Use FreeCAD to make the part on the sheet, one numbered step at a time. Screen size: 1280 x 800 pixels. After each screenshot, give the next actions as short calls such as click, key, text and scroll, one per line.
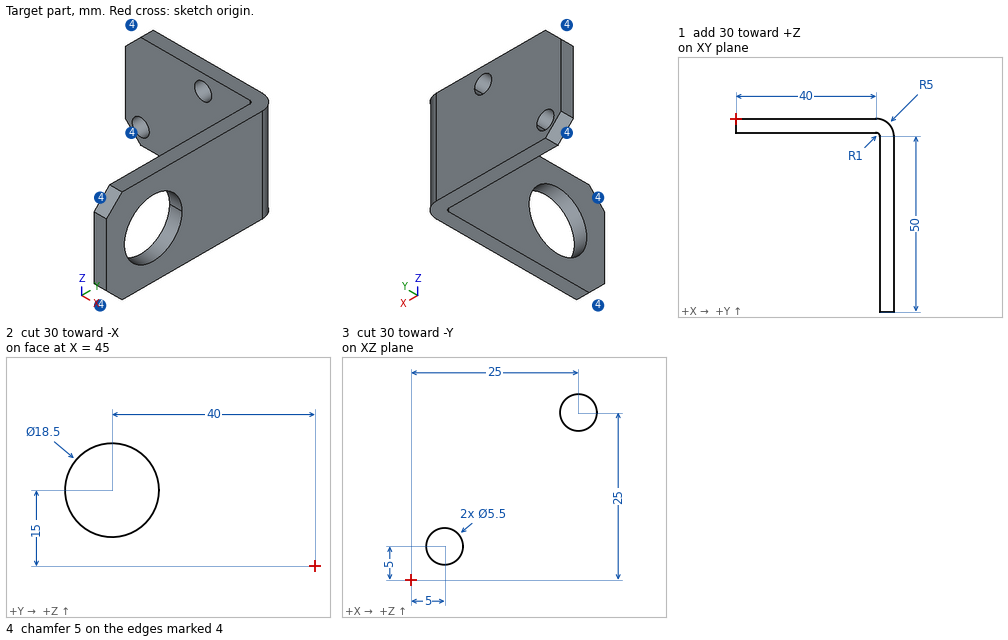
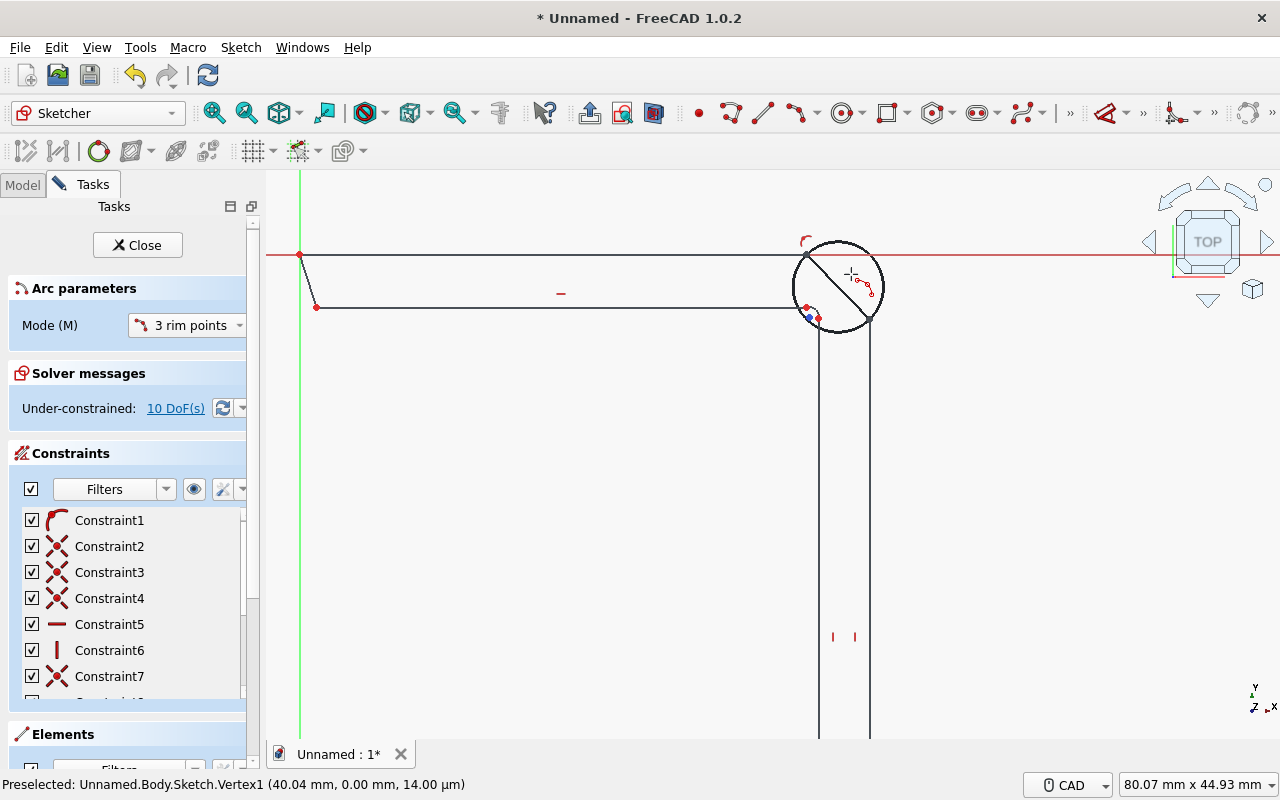
click(851, 273)
key(Escape)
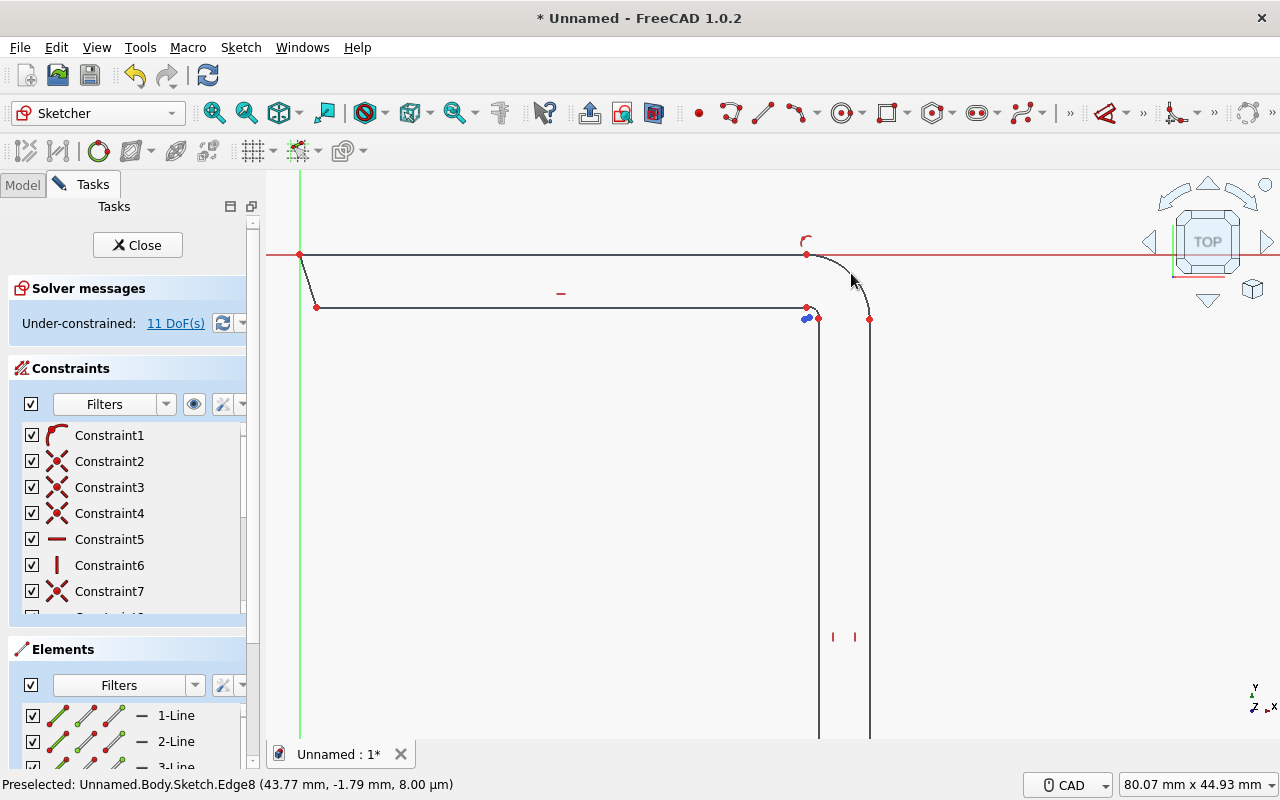
click(655, 255)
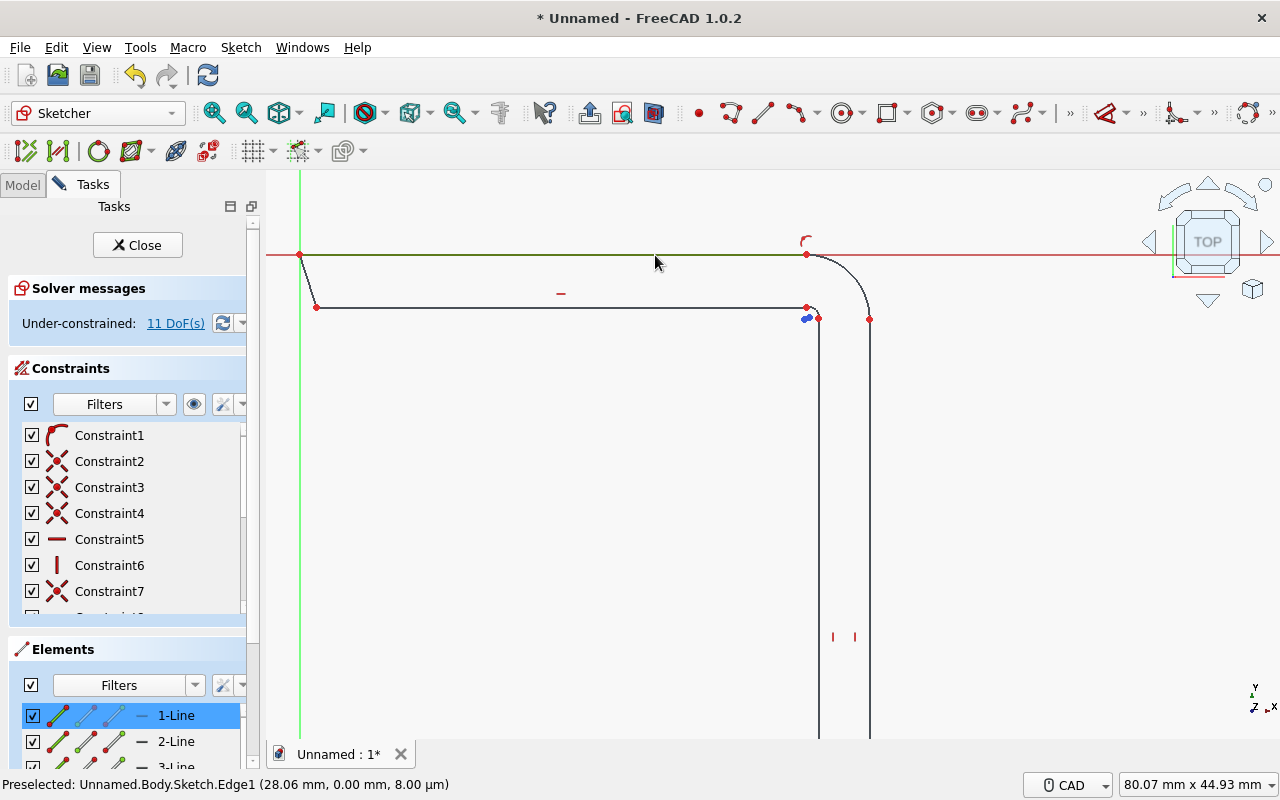
click(863, 291)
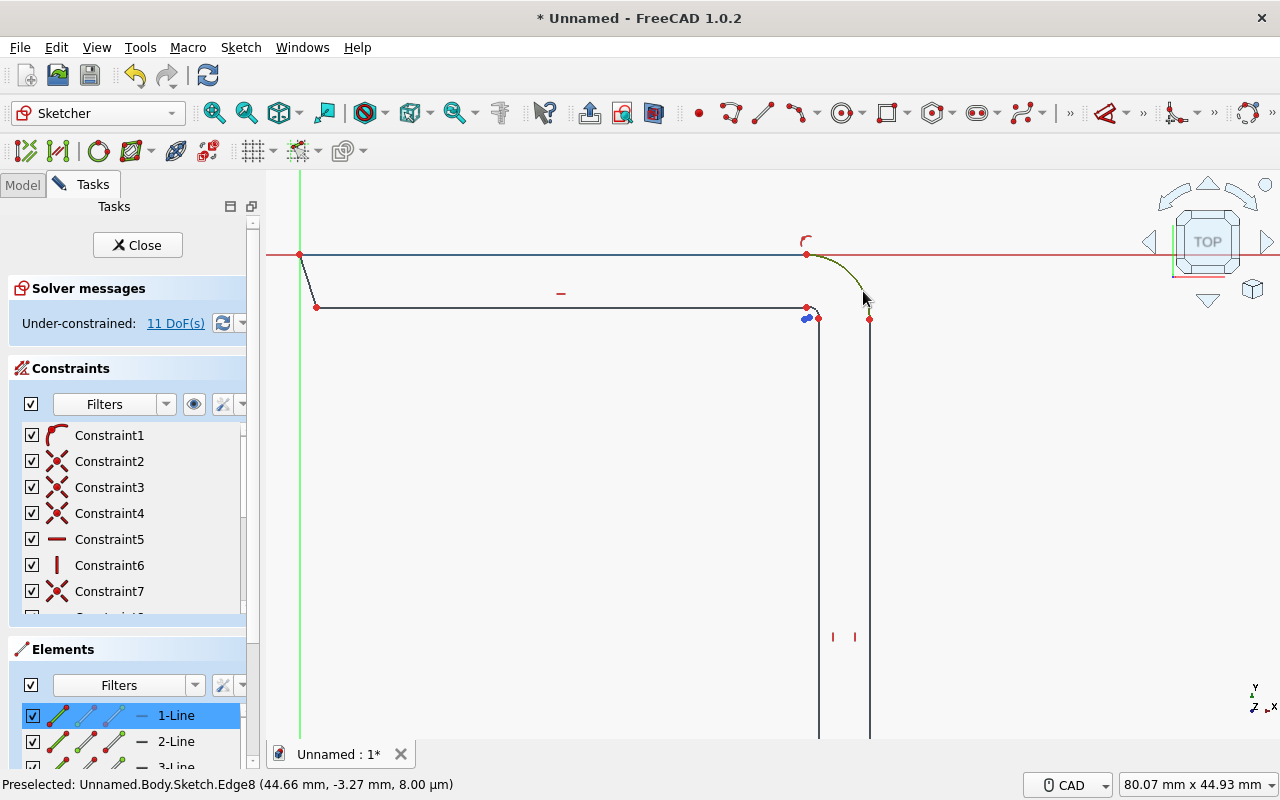
key(t)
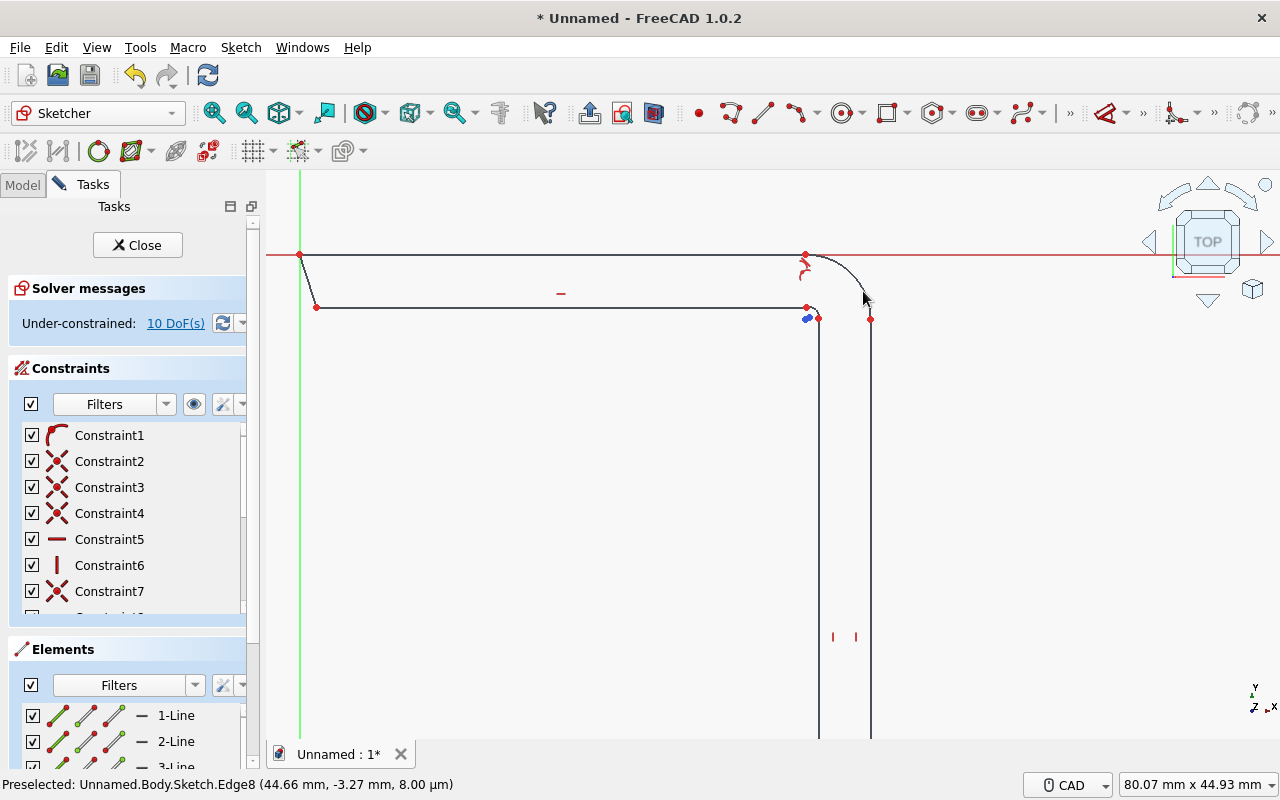
click(464, 308)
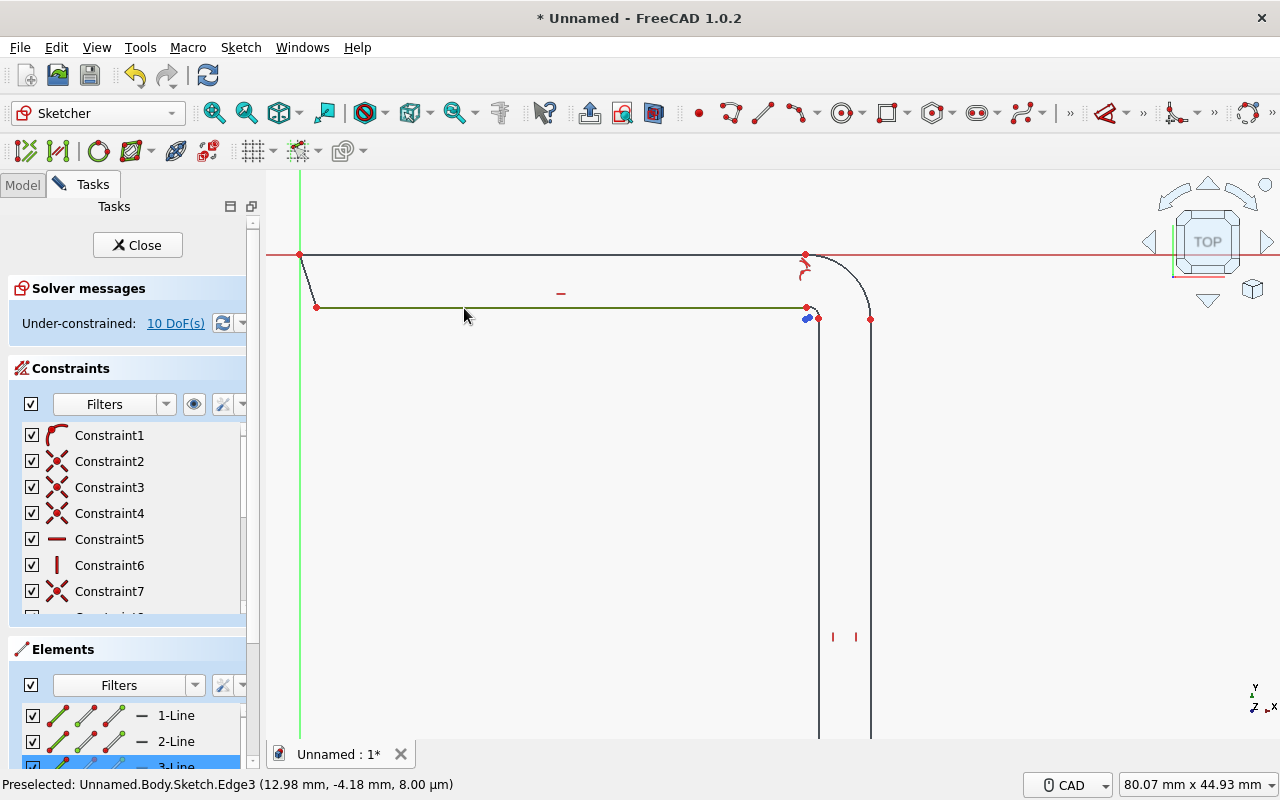
scroll(816, 310, up, 2)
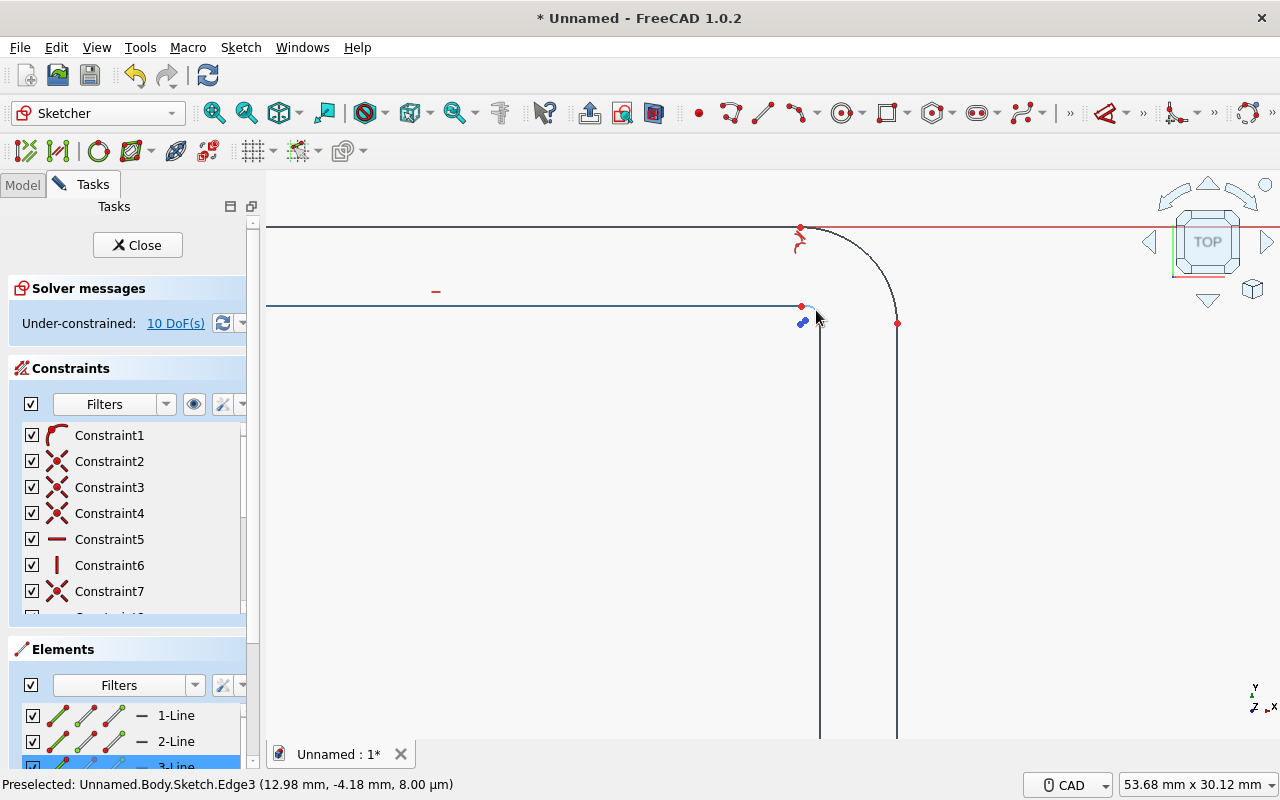
click(815, 310)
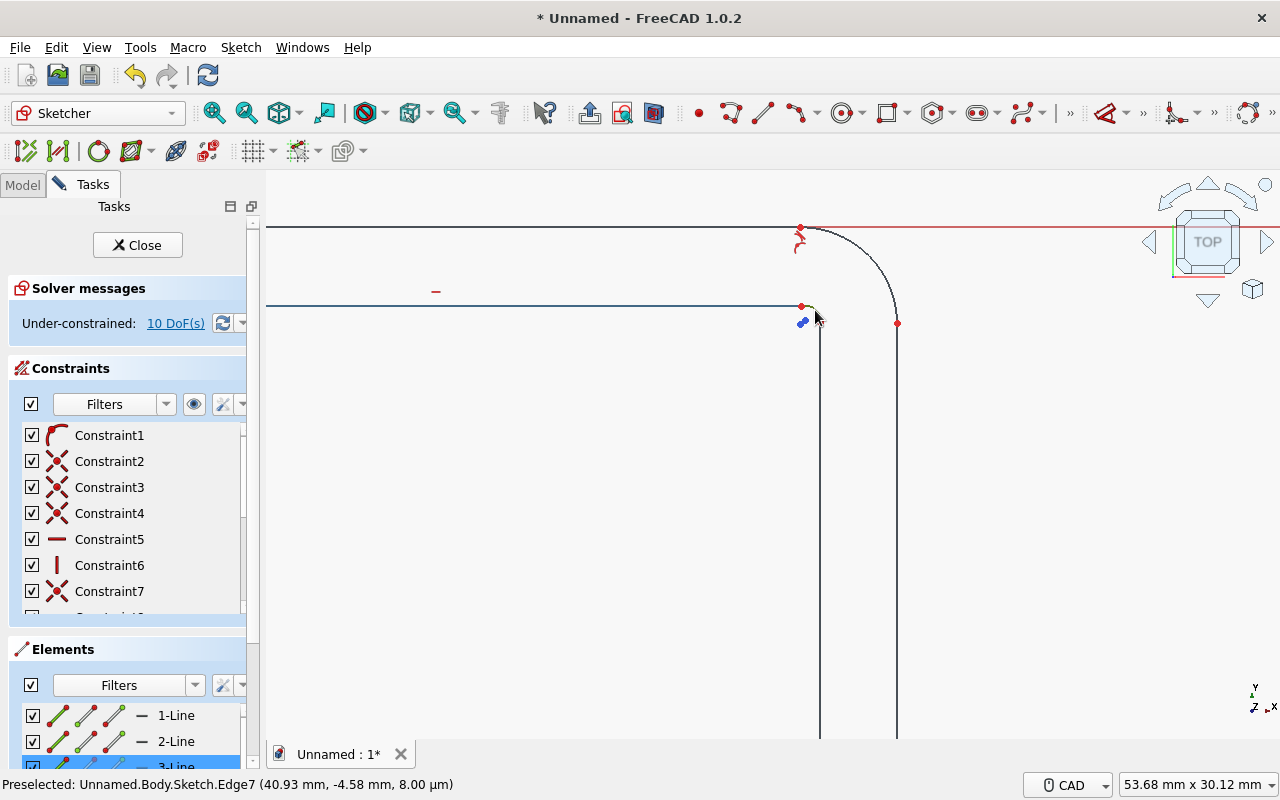
key(t)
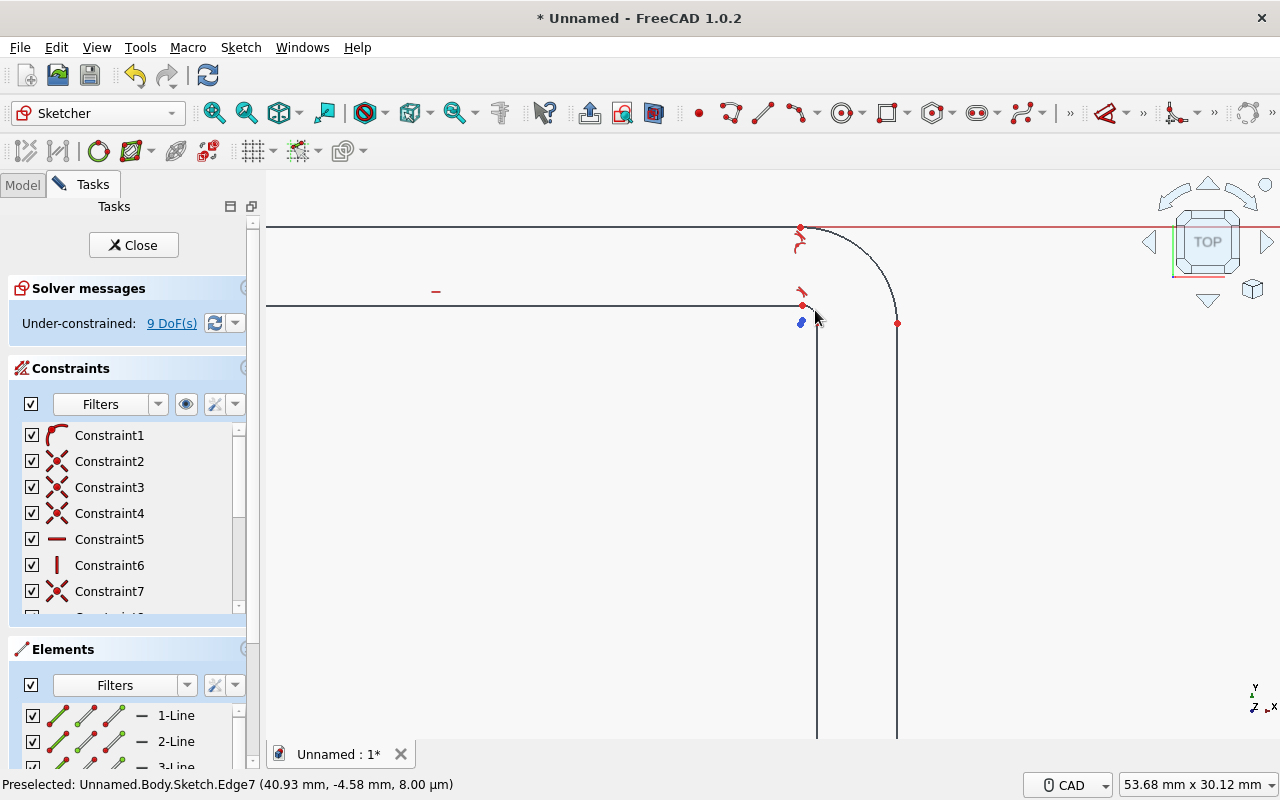
click(817, 607)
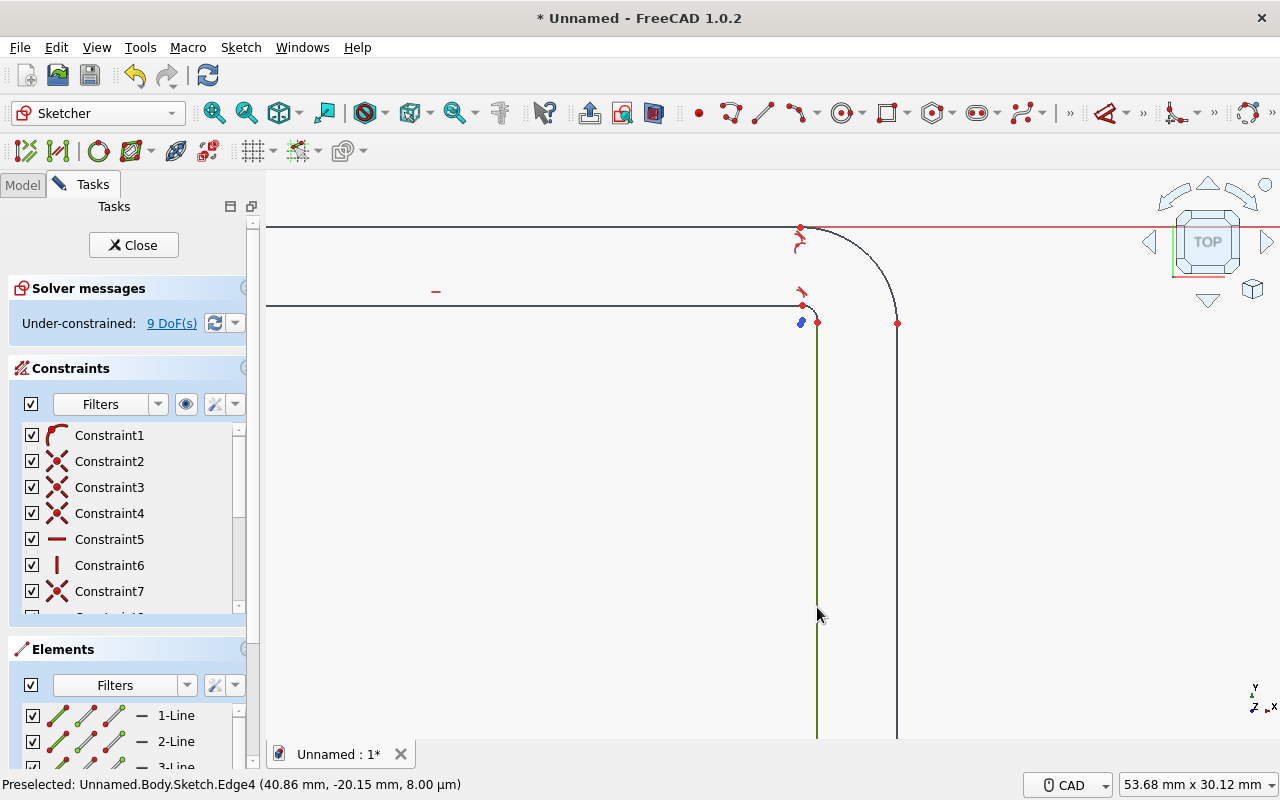
click(814, 311)